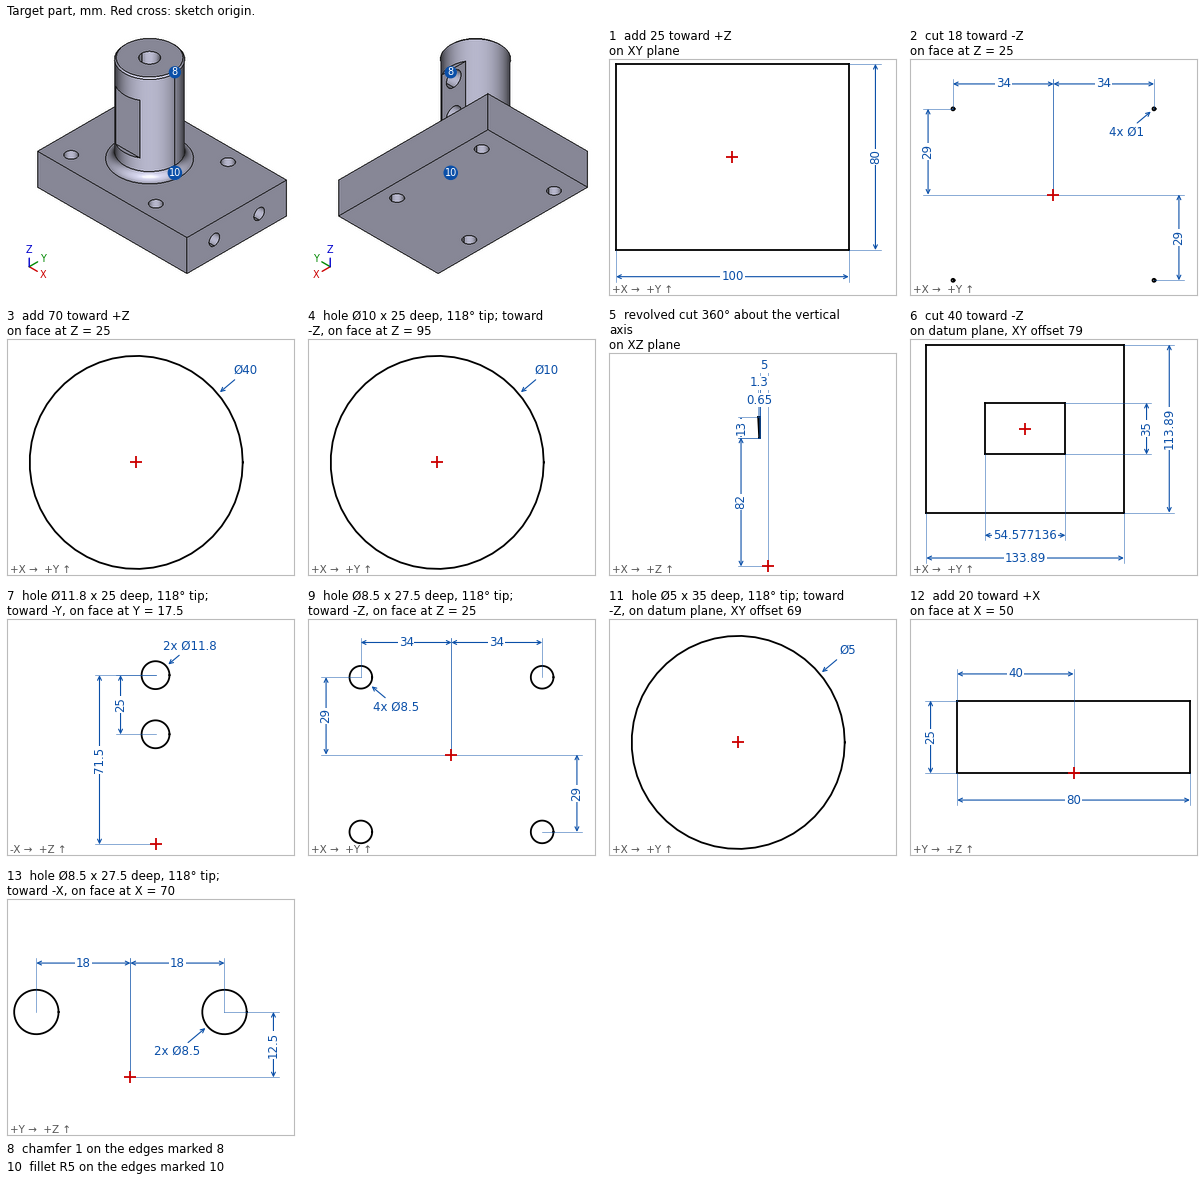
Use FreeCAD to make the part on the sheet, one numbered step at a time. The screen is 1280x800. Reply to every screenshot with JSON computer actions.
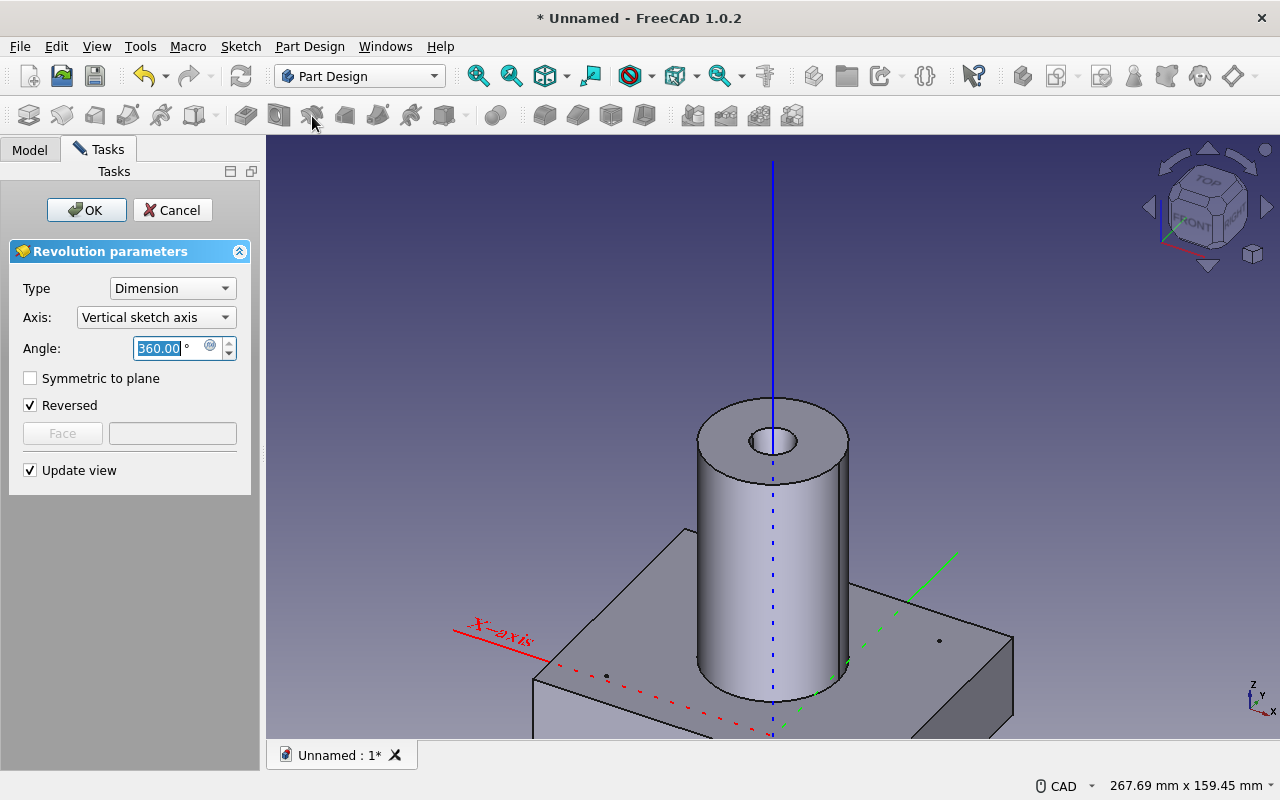
{"action": "left_click", "coordinate": [87, 210]}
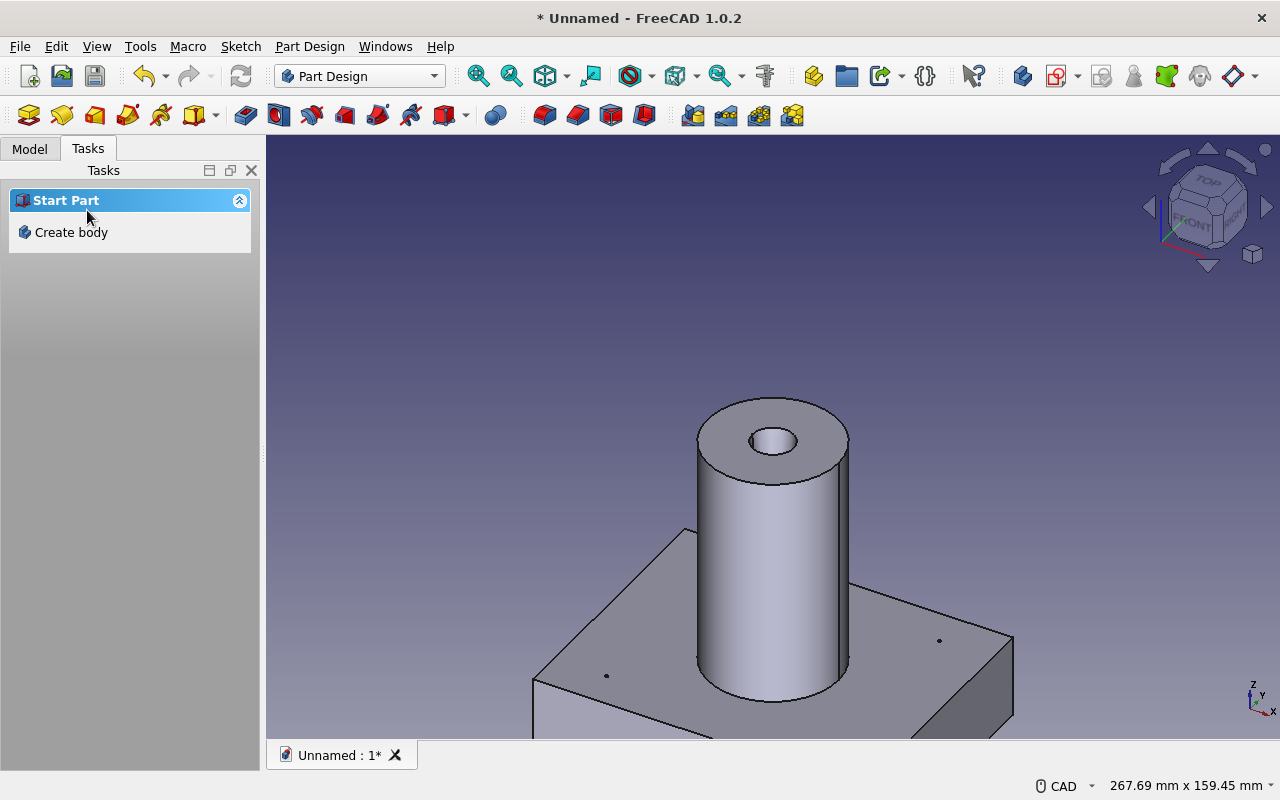
{"action": "key", "text": "v f"}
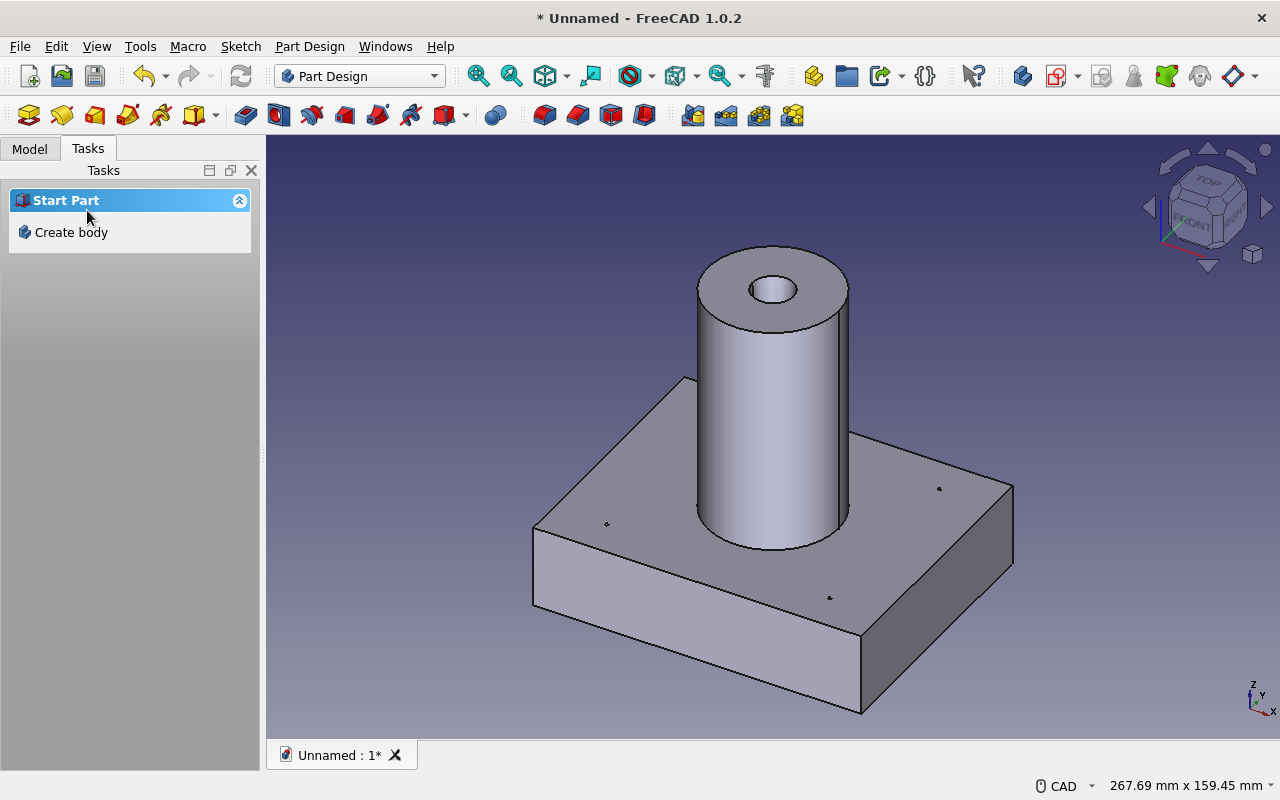
{"action": "left_click", "coordinate": [30, 148]}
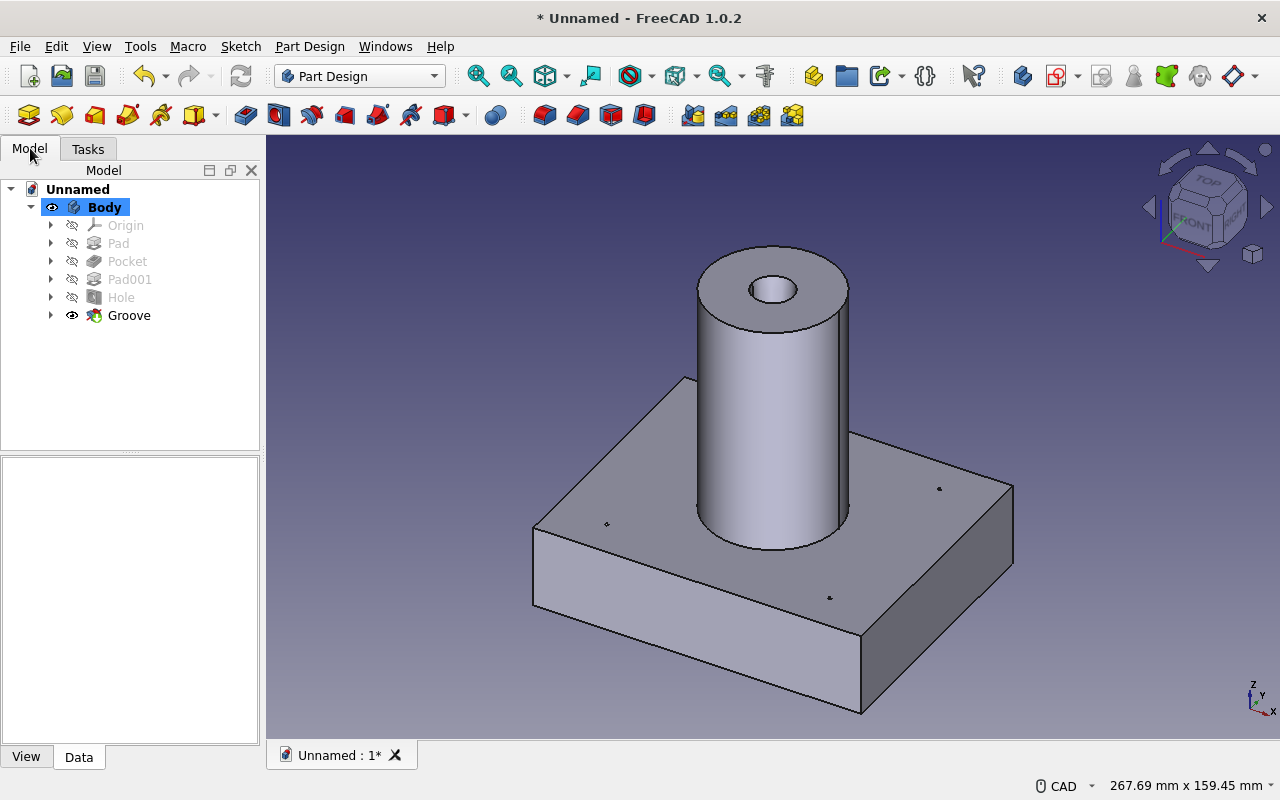
{"action": "left_click", "coordinate": [51, 225]}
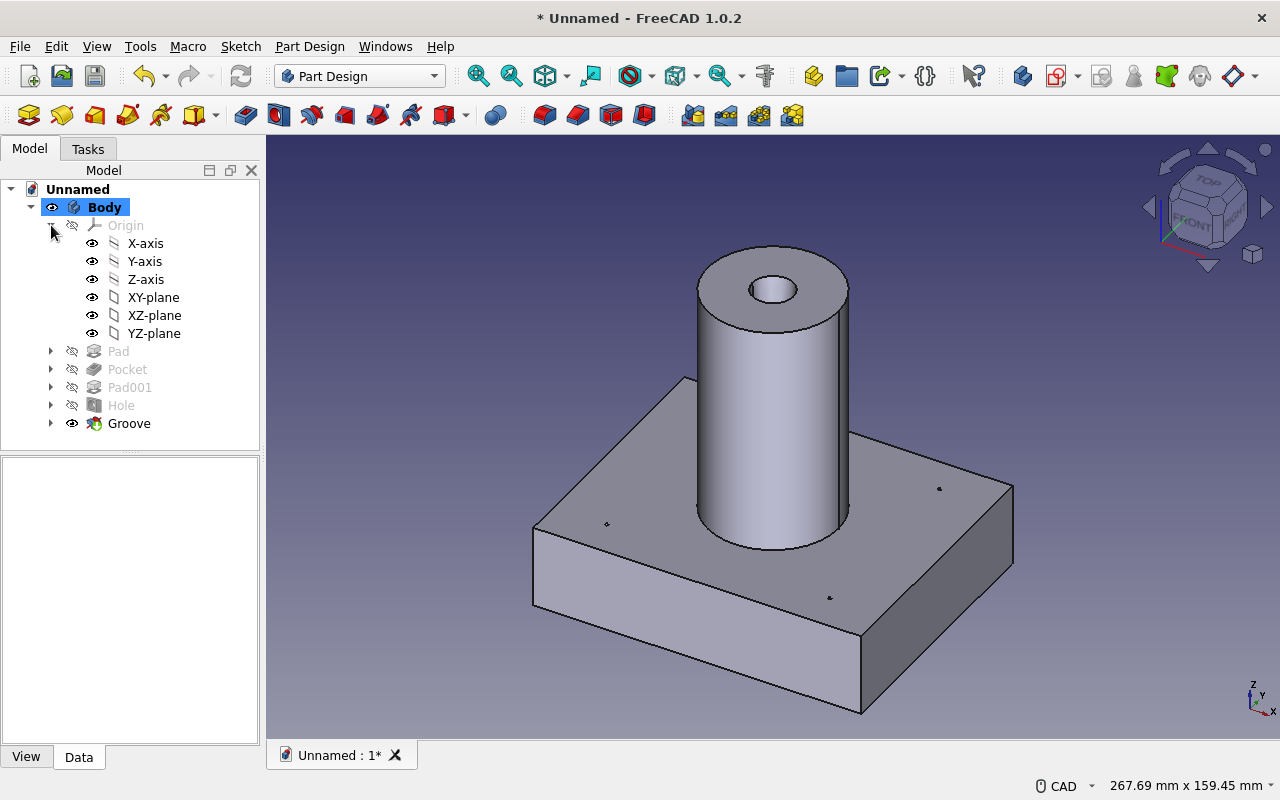
{"action": "left_click", "coordinate": [137, 297]}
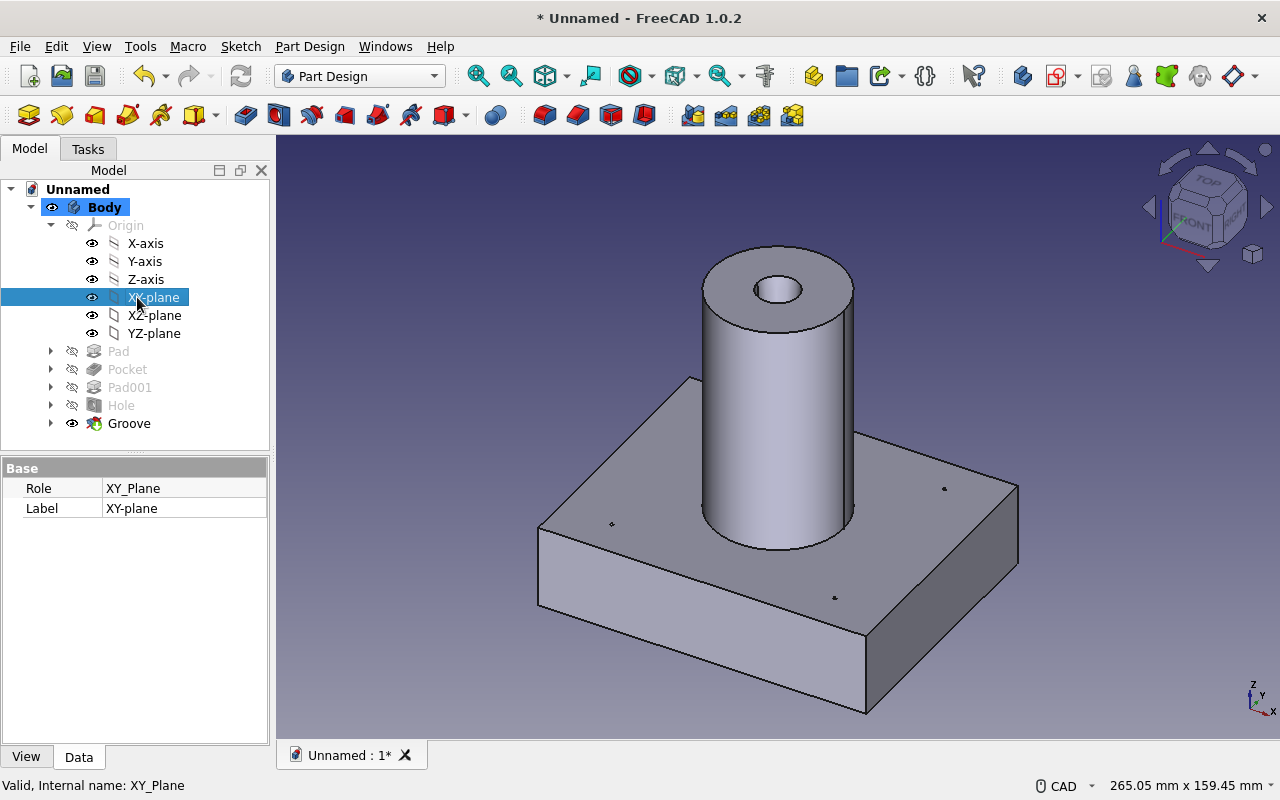
{"action": "left_click", "coordinate": [1232, 76]}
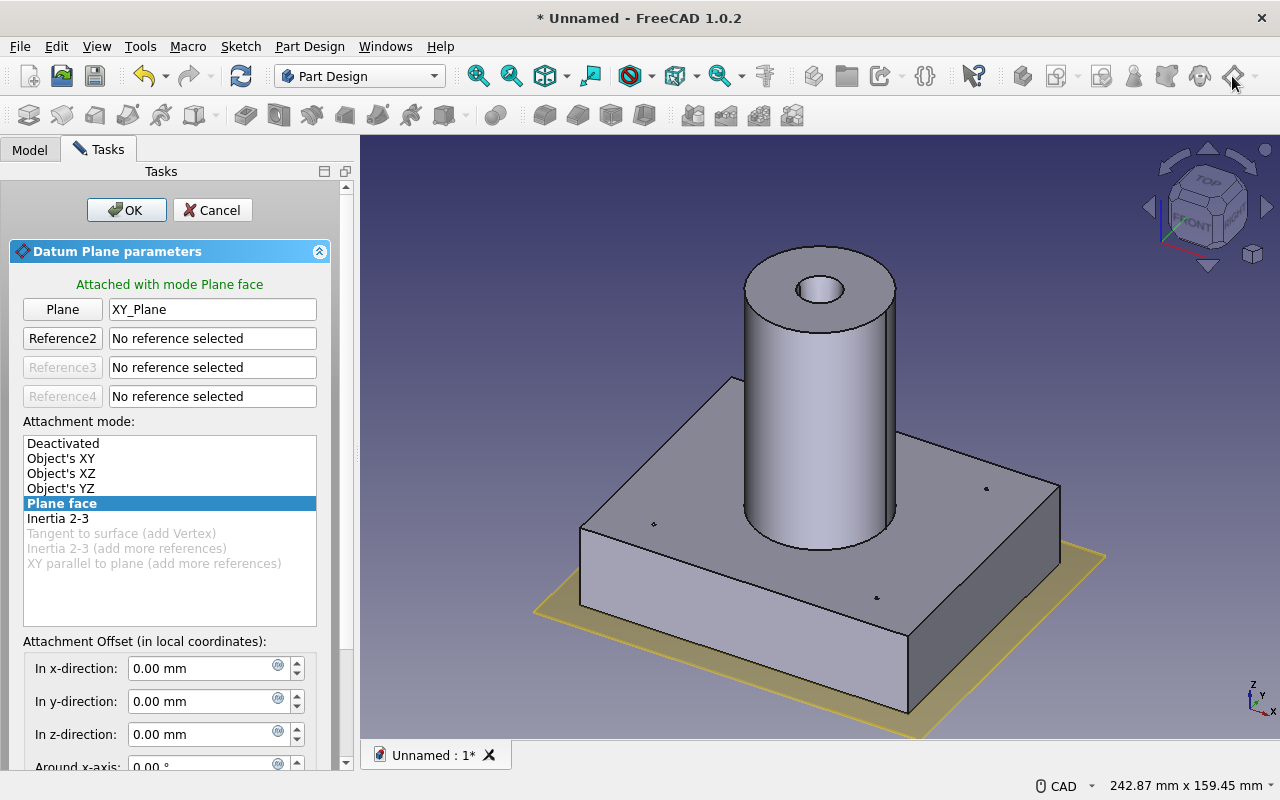
{"action": "triple_click", "coordinate": [210, 734]}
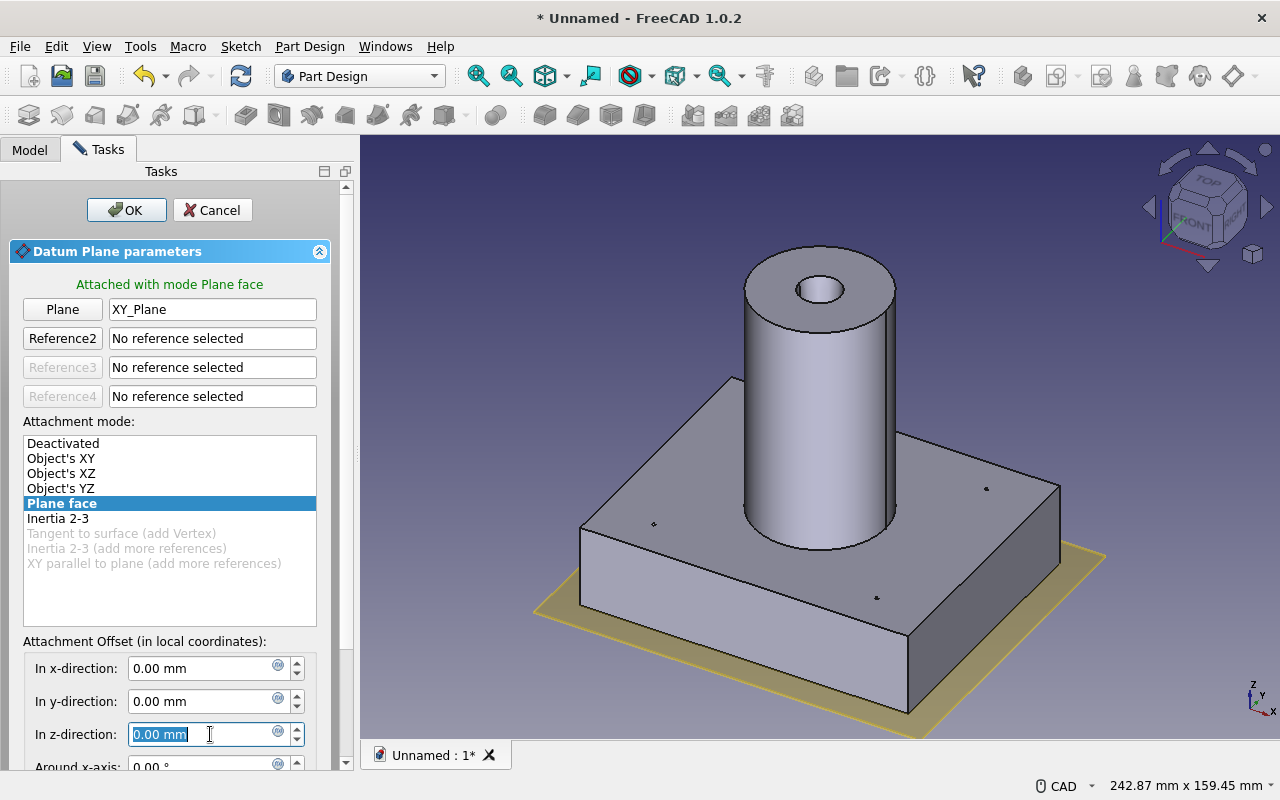
{"action": "type", "text": "79"}
{"action": "key", "text": "Tab"}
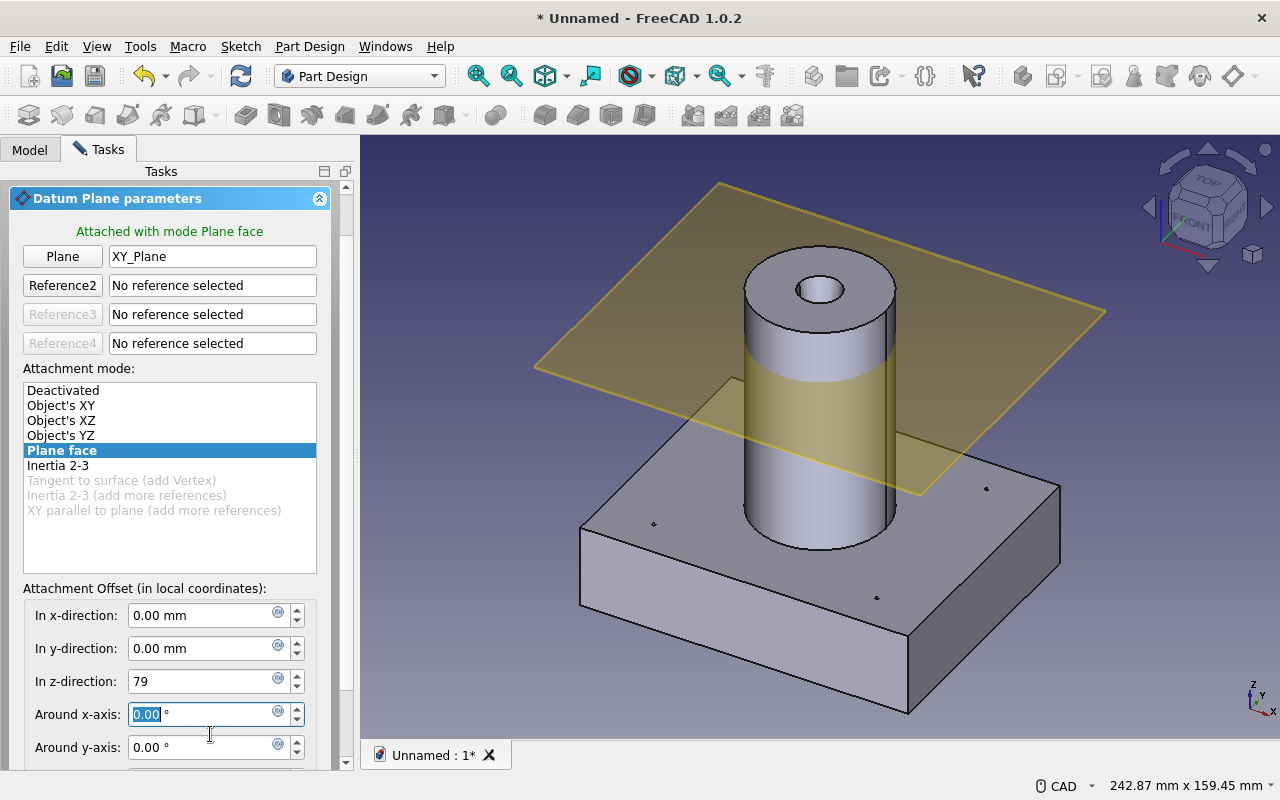
{"action": "scroll", "coordinate": [346, 476], "scroll_direction": "up", "scroll_amount": 2}